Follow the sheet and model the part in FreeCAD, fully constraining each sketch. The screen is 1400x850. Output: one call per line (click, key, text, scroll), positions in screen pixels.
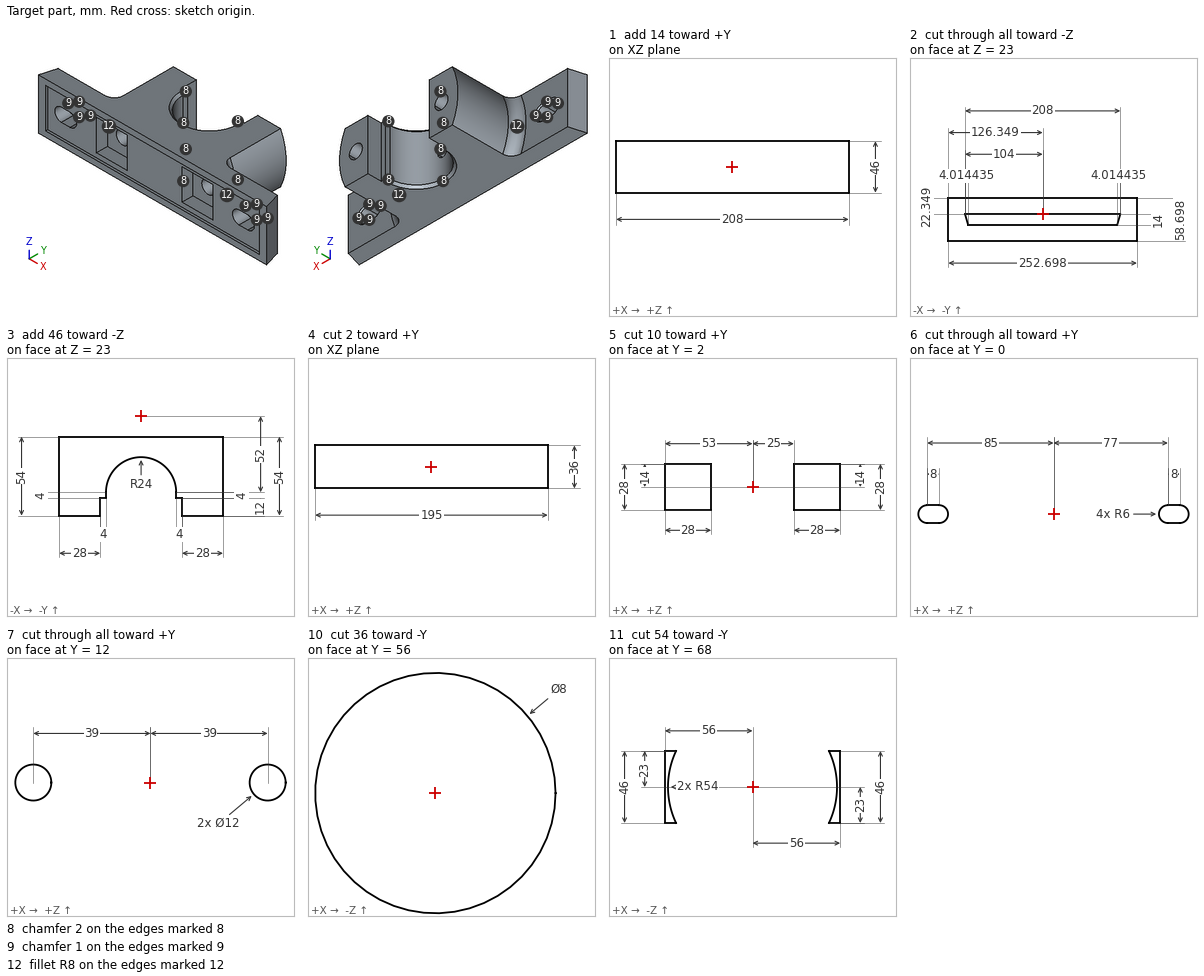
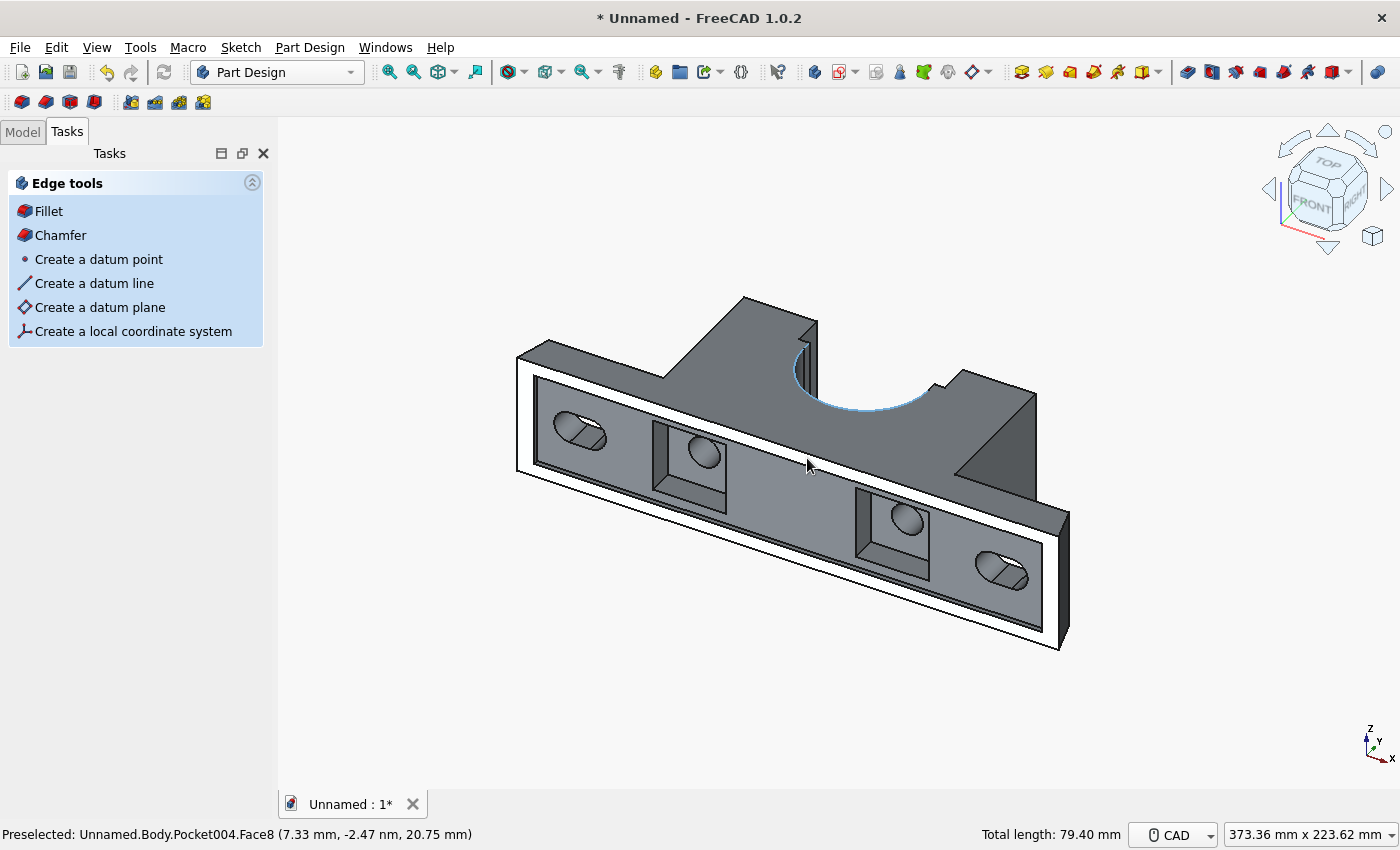
key(0)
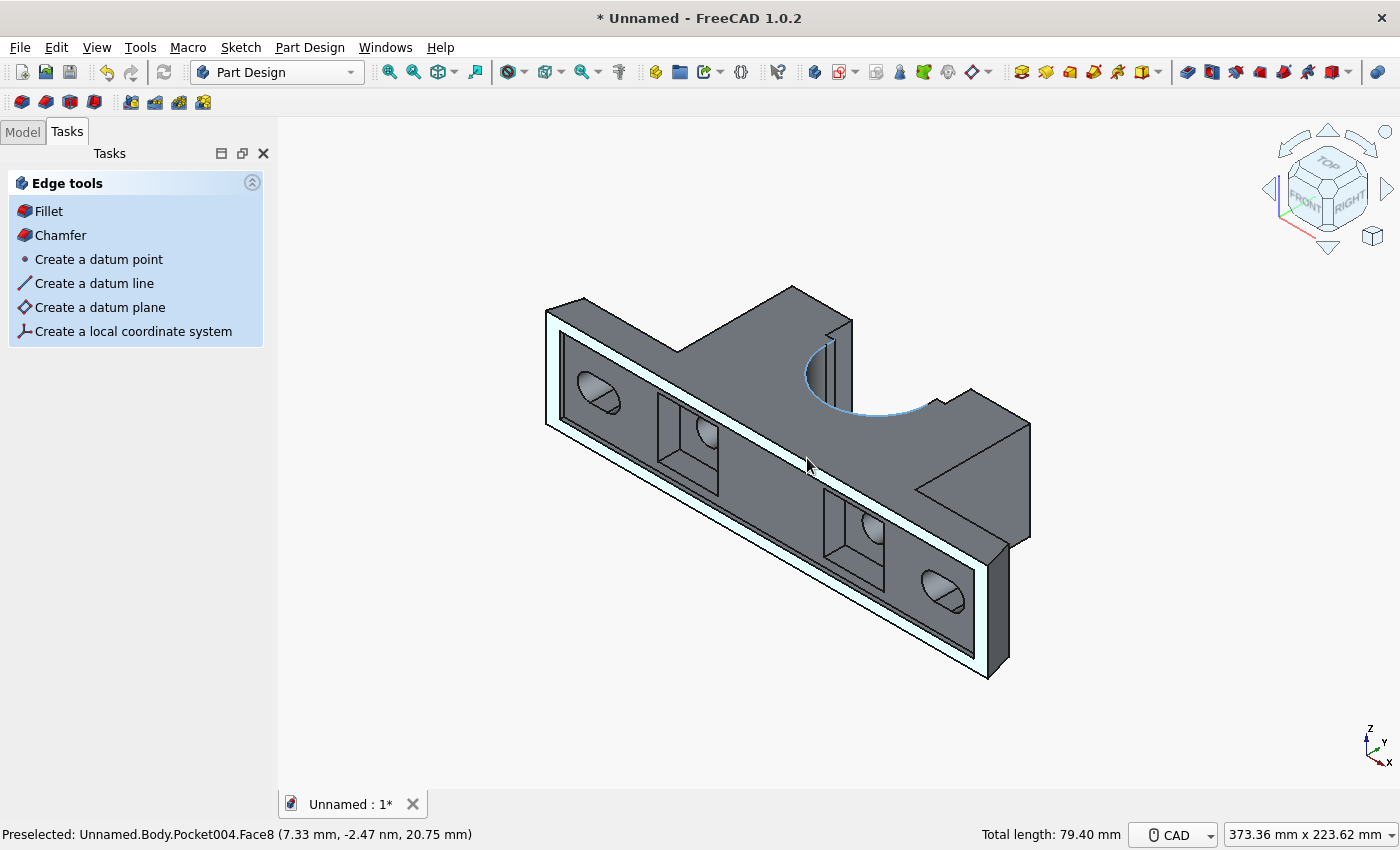
scroll(831, 454, up, 7)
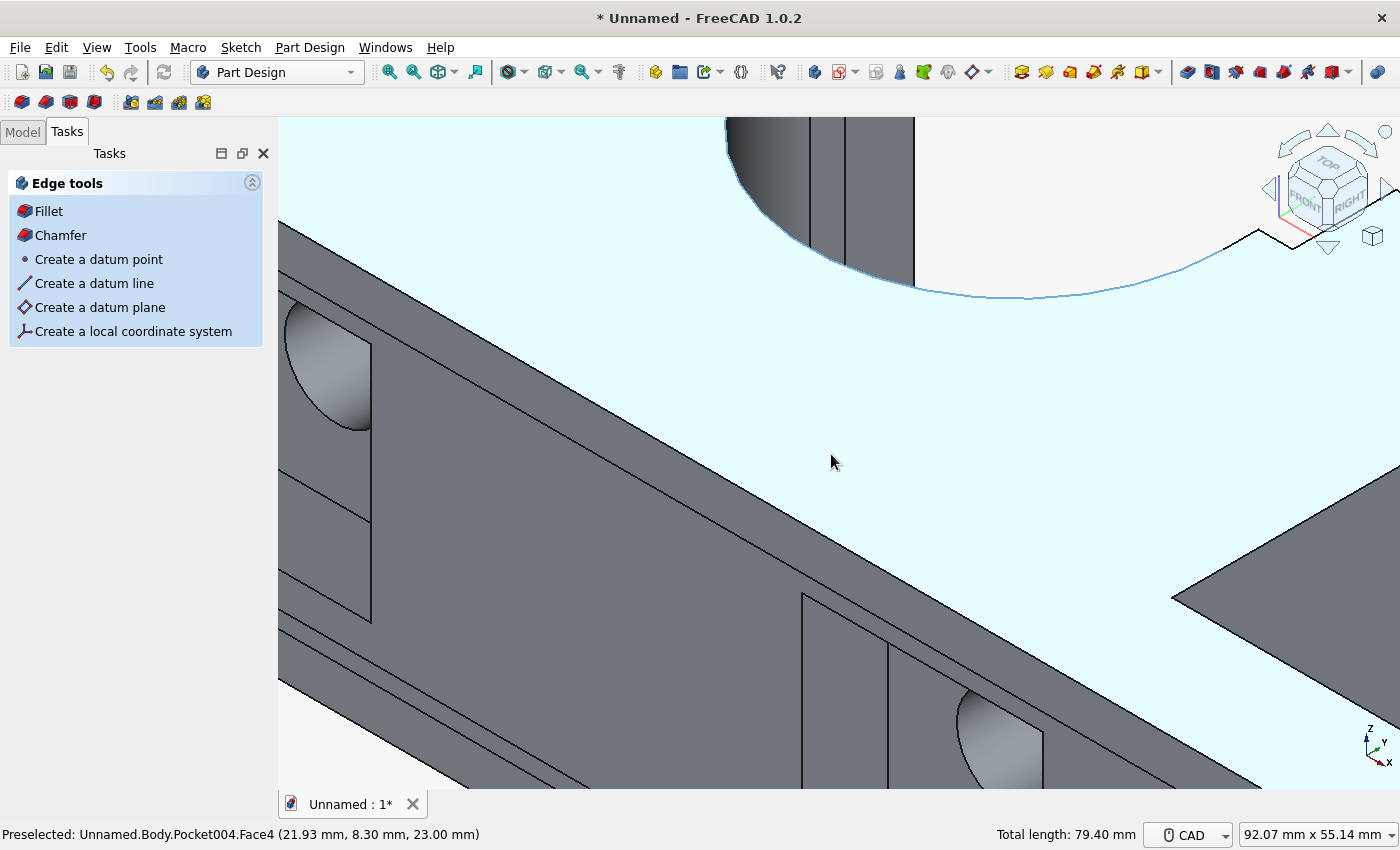
click(390, 72)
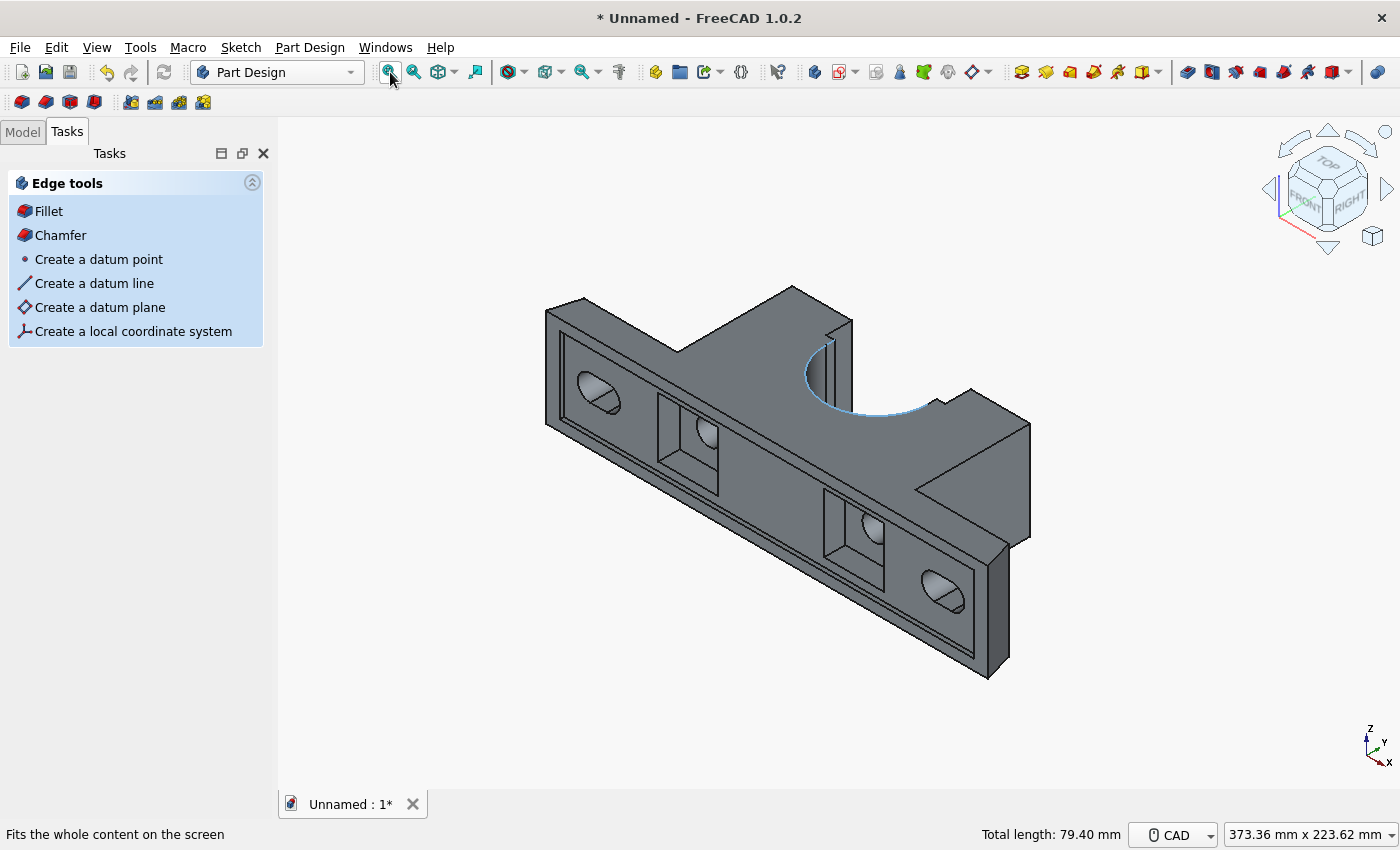
key(2)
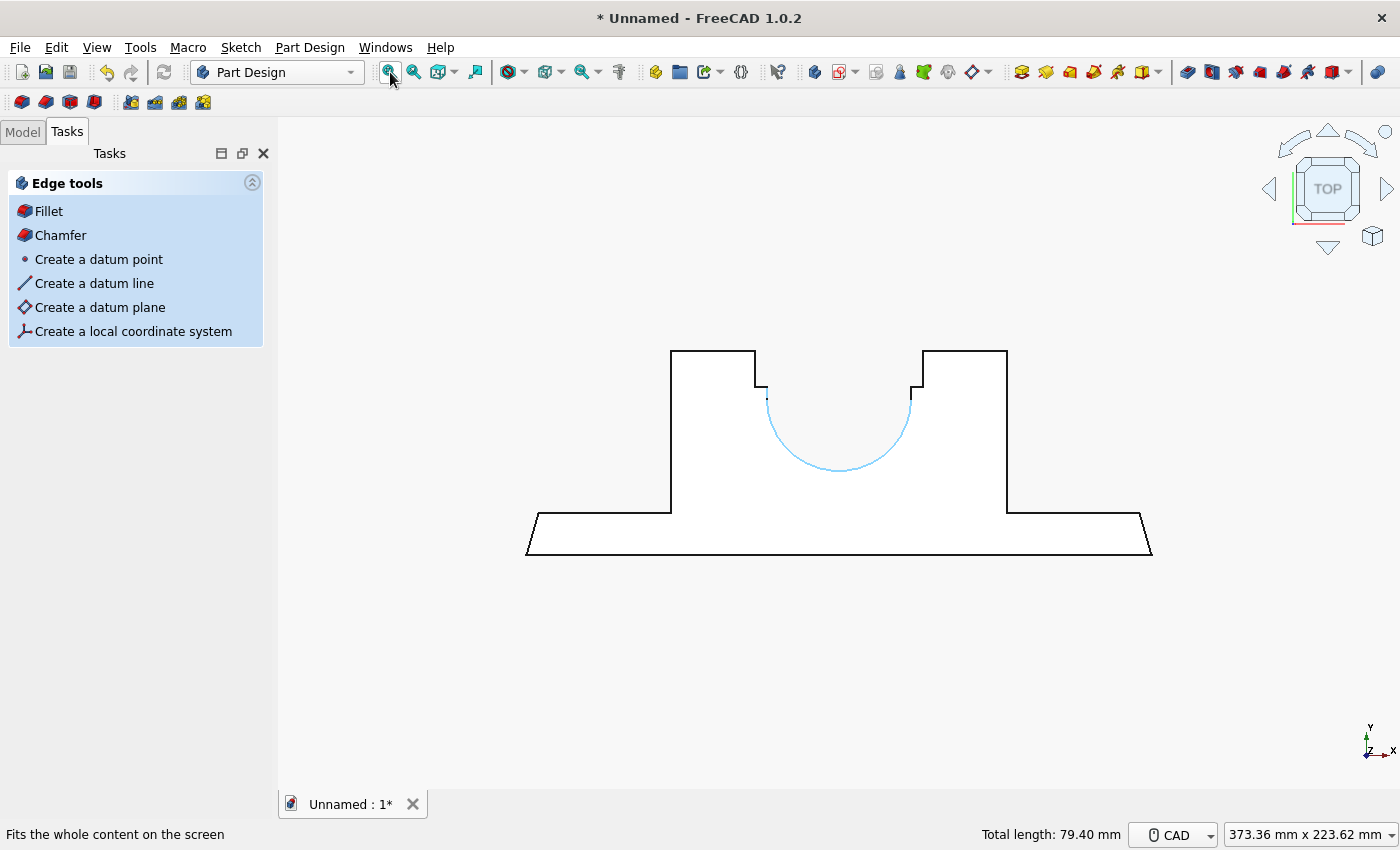
click(911, 392, ctrl)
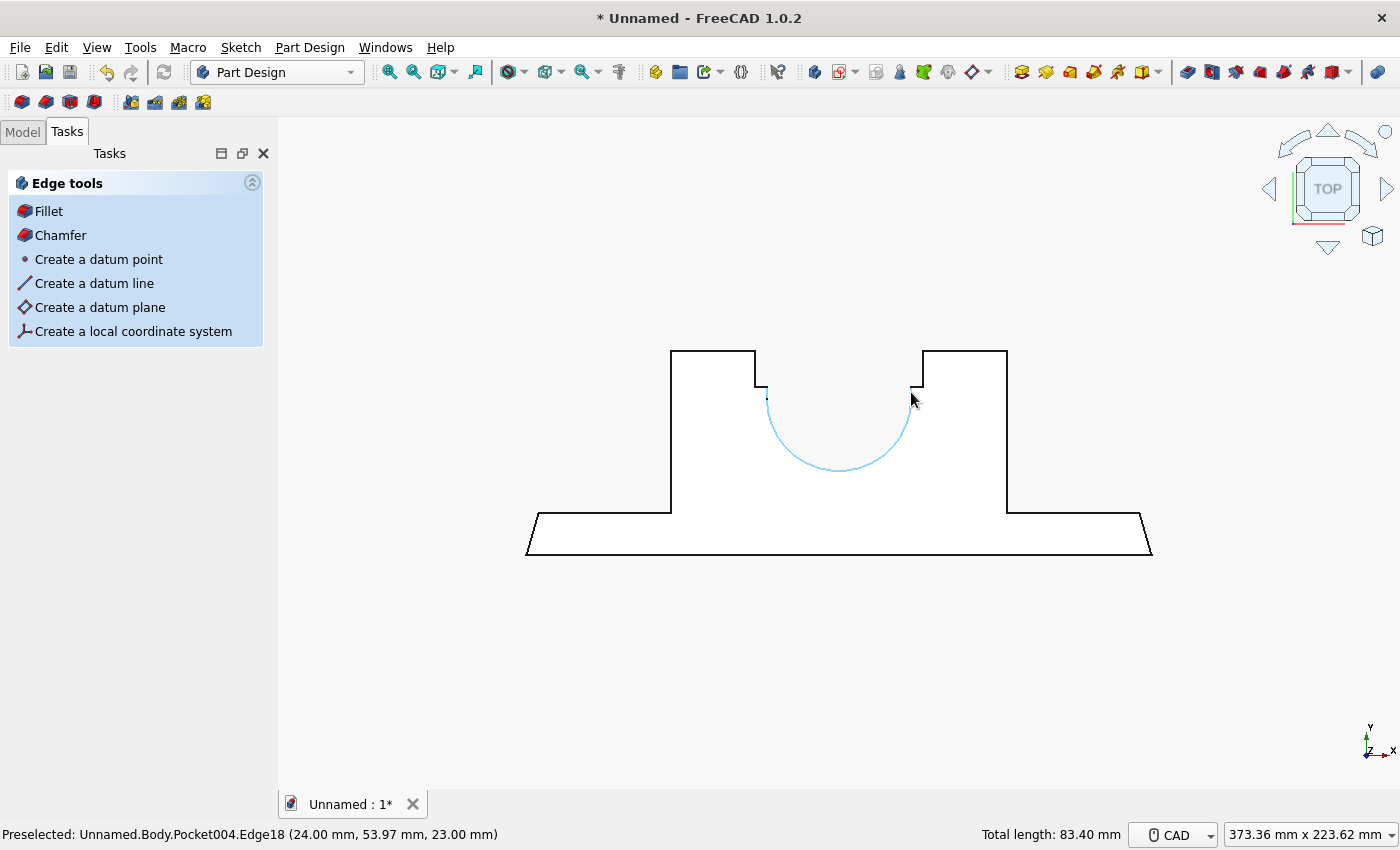
scroll(767, 392, up, 7)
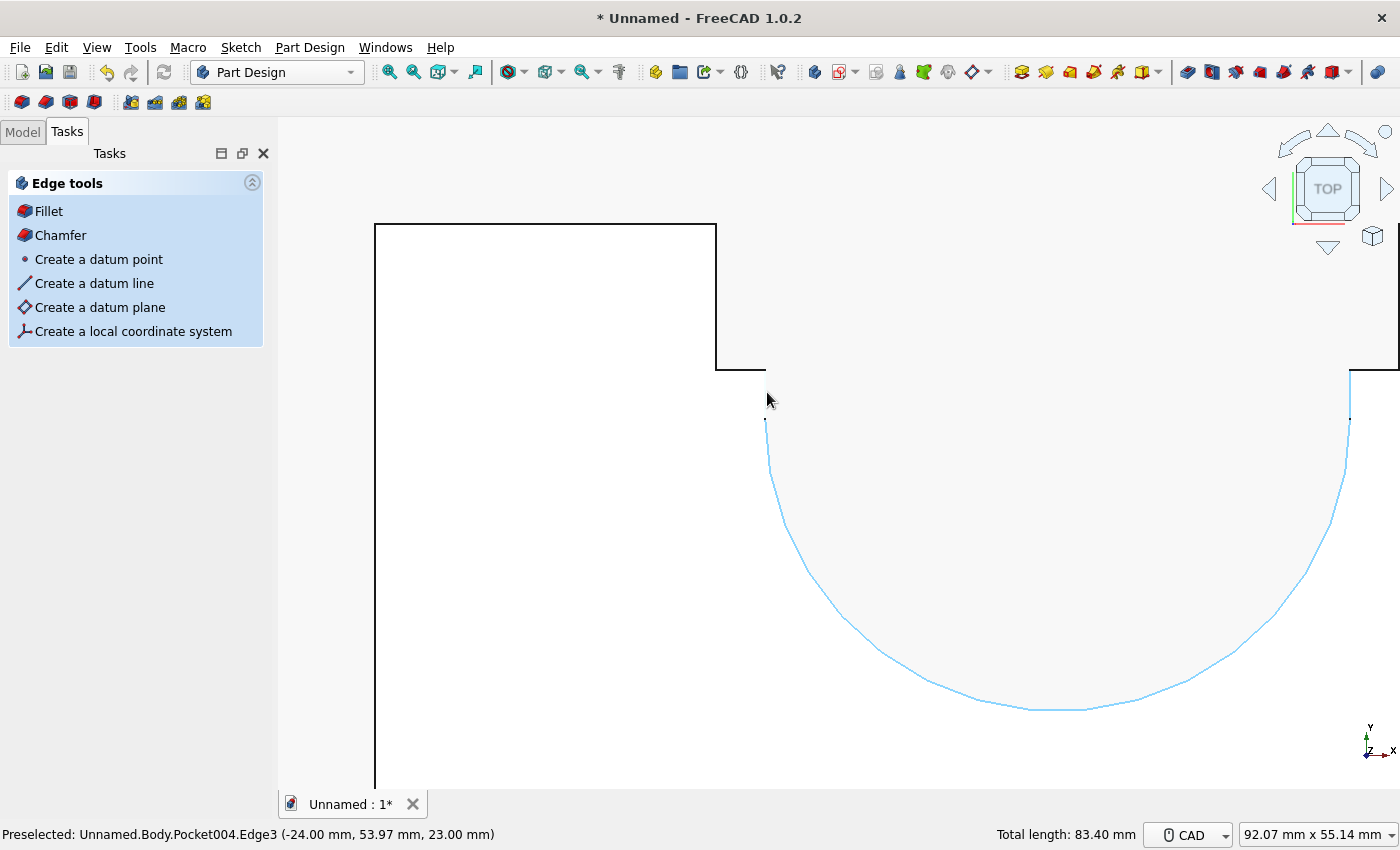
key(v)
key(f)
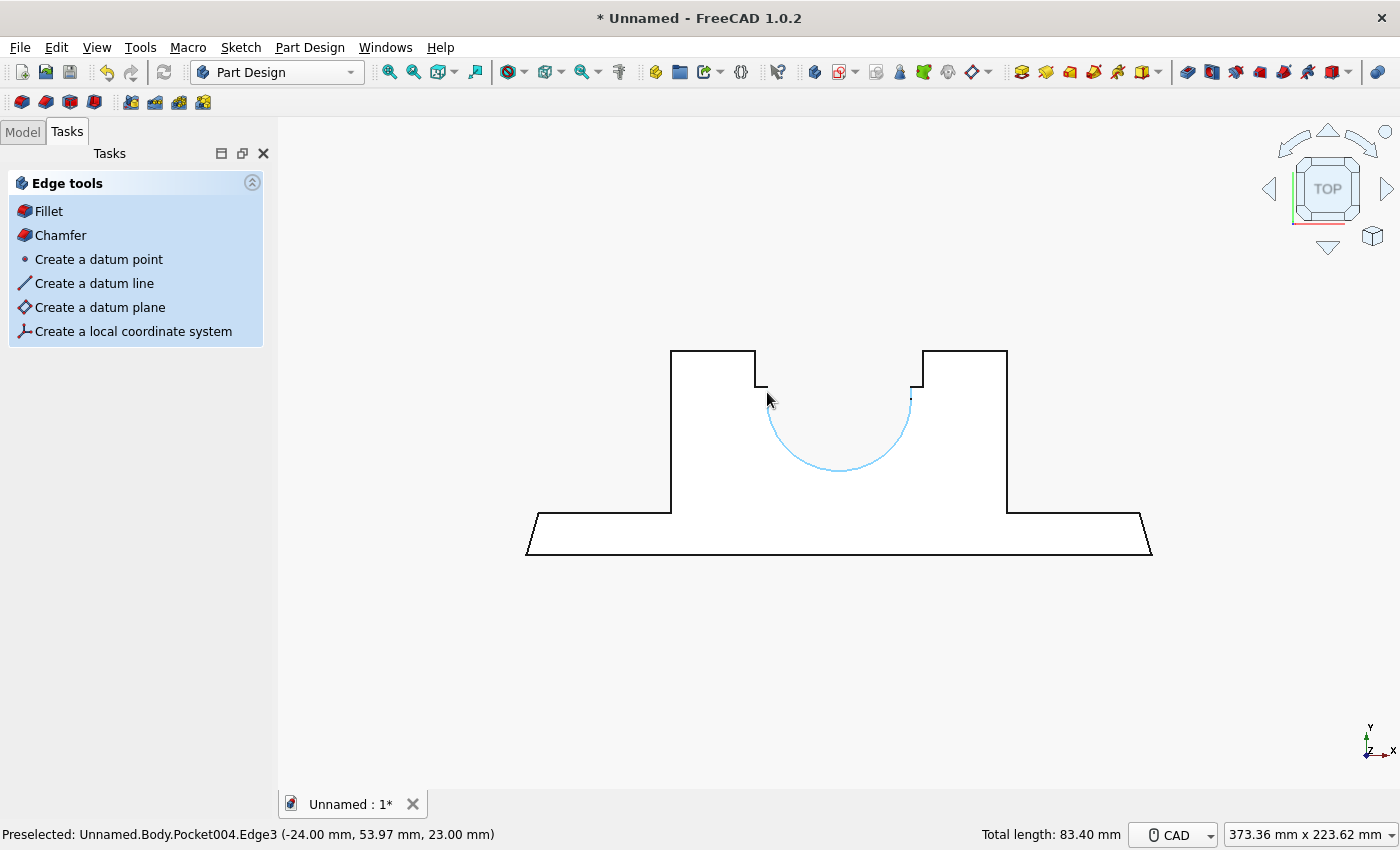
key(1)